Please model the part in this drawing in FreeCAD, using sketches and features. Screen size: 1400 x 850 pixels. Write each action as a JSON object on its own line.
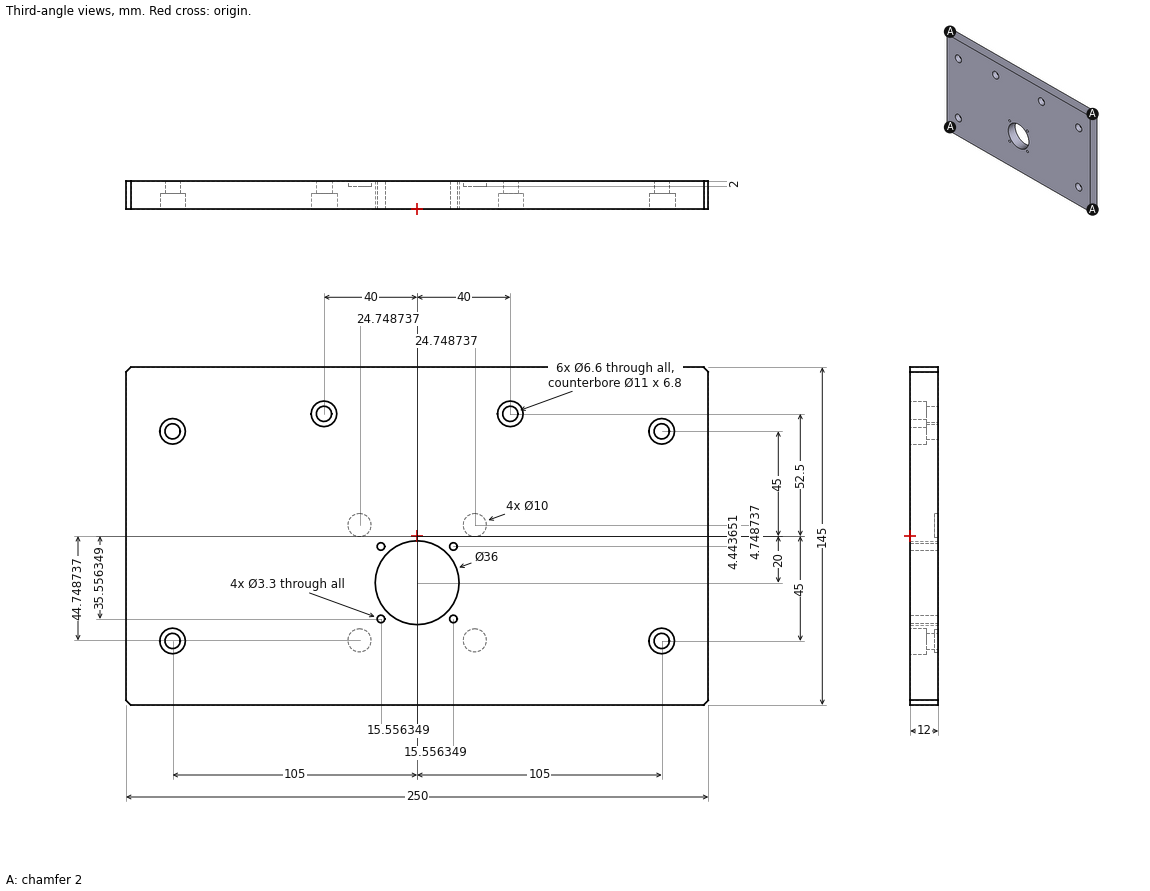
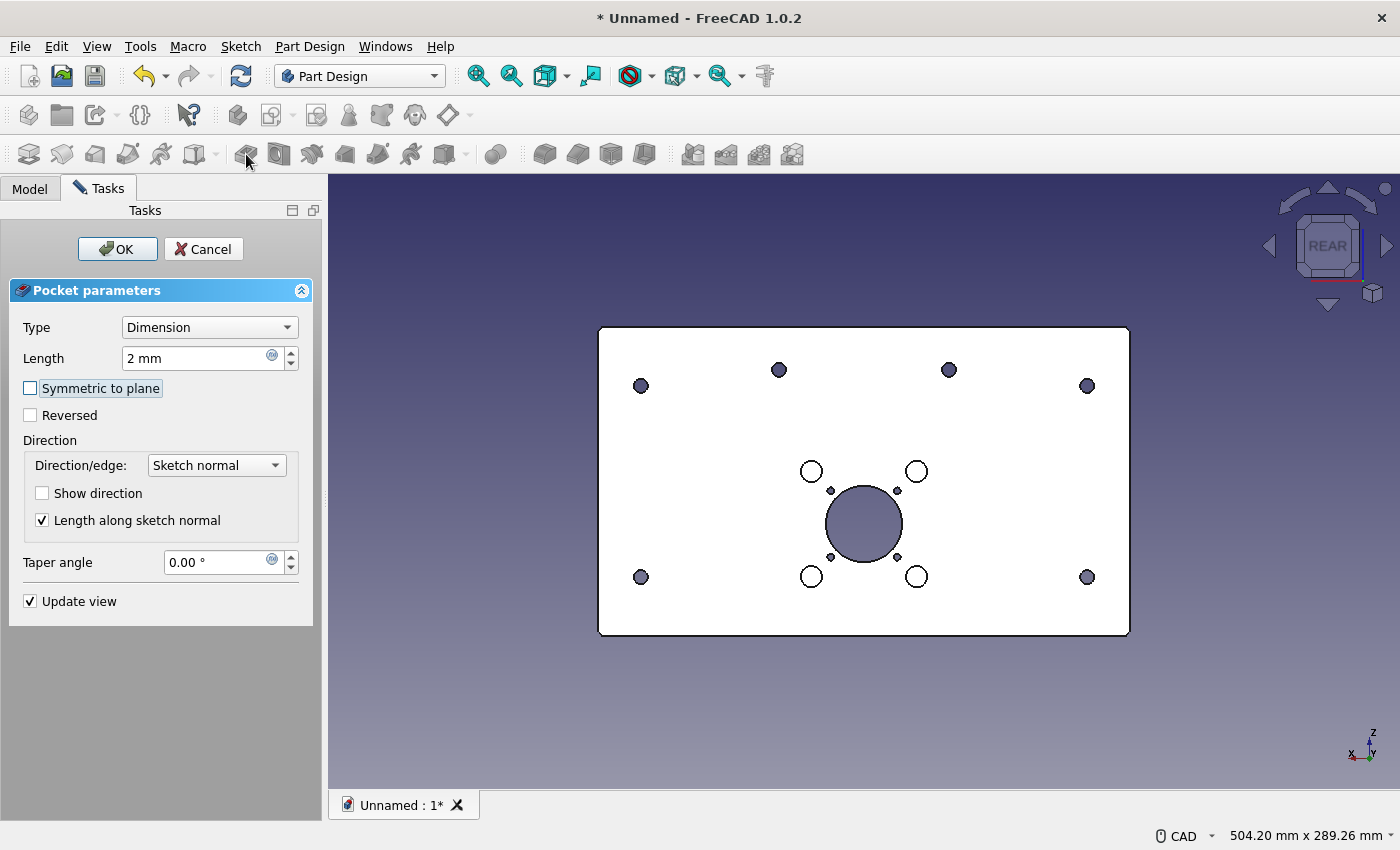
{"action": "left_click", "coordinate": [118, 249]}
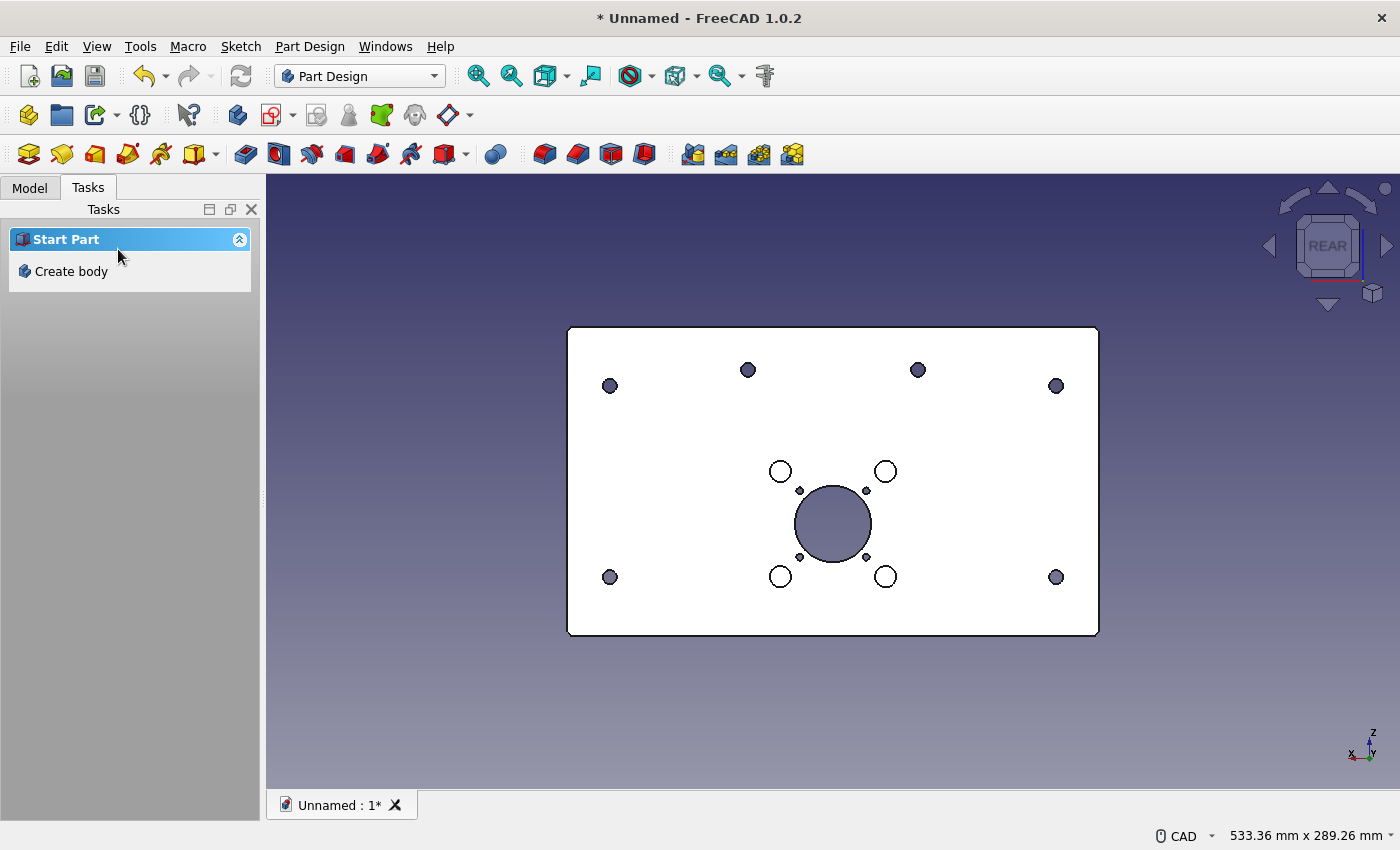
{"action": "key", "text": "0"}